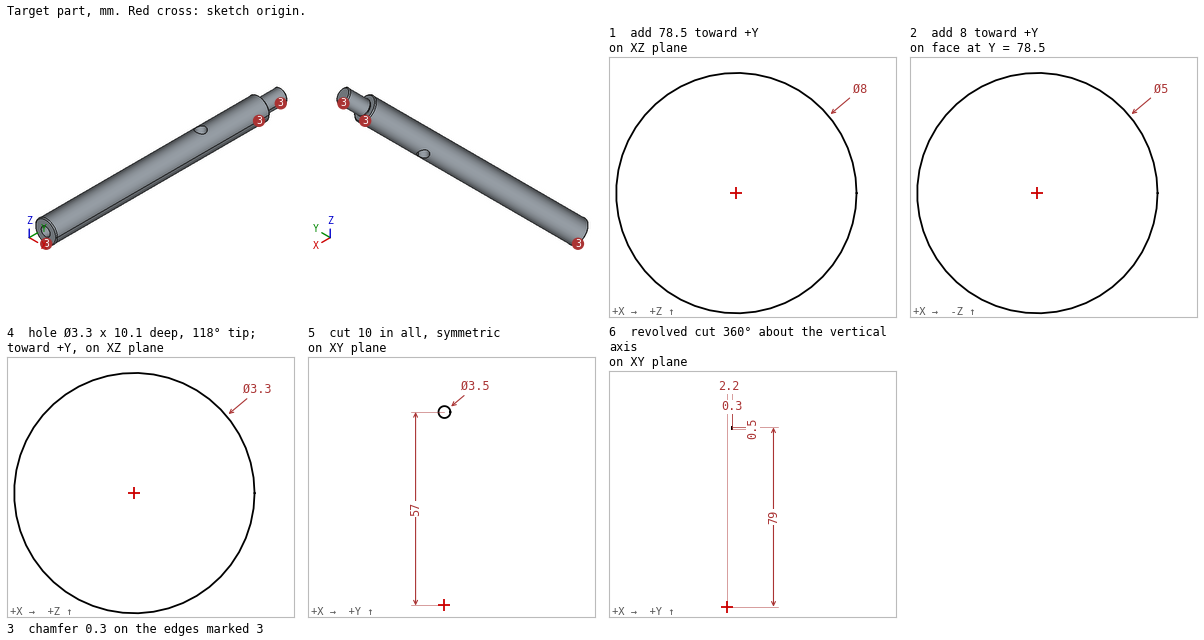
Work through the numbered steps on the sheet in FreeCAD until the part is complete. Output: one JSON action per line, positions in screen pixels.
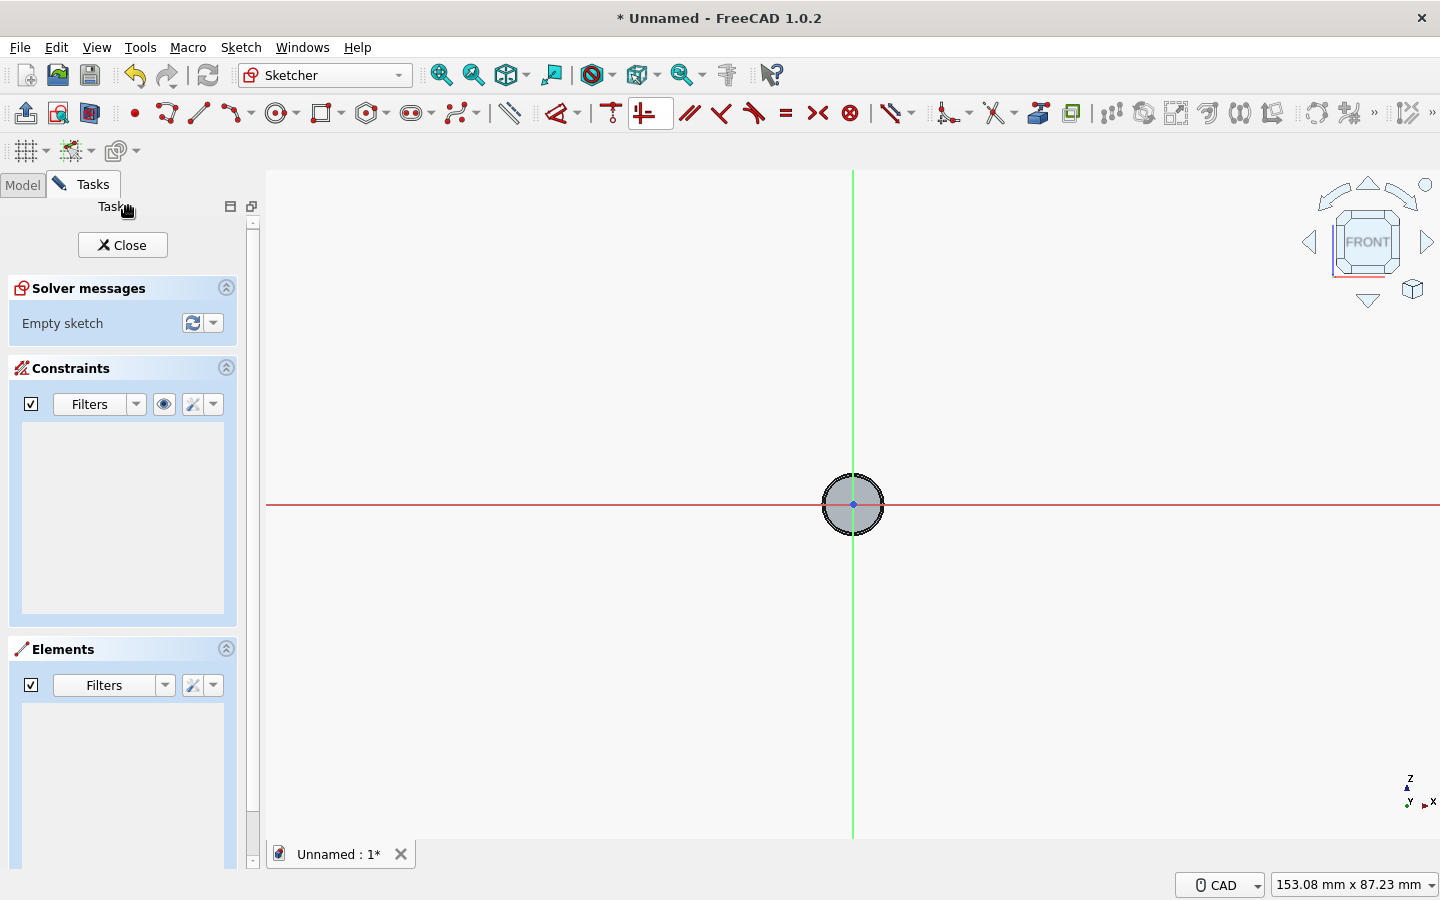
{"action": "scroll", "coordinate": [857, 505], "scroll_direction": "up", "scroll_amount": 14}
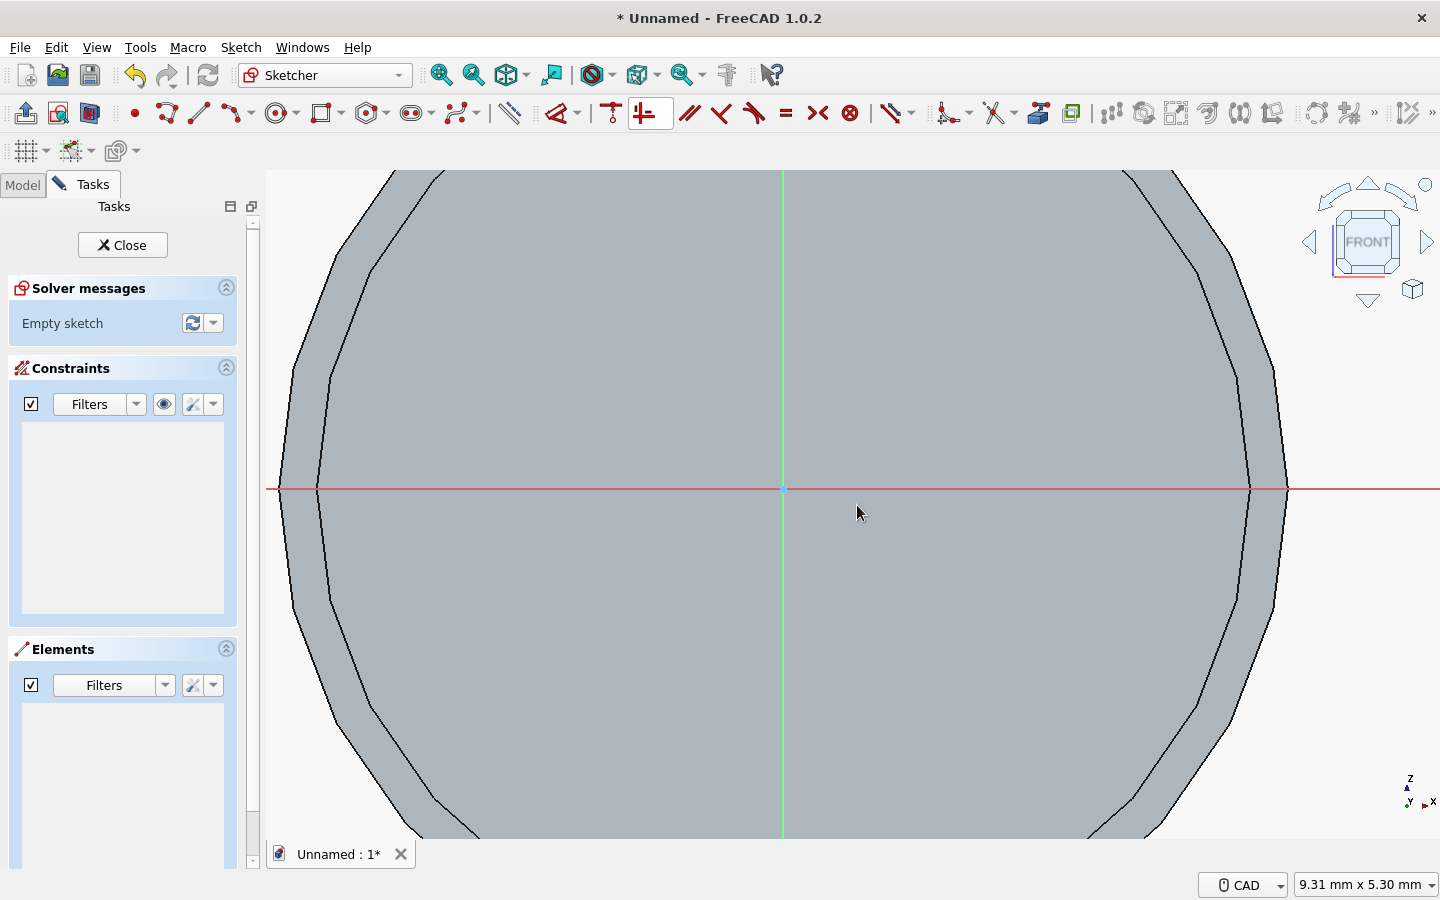
{"action": "key", "text": "g c"}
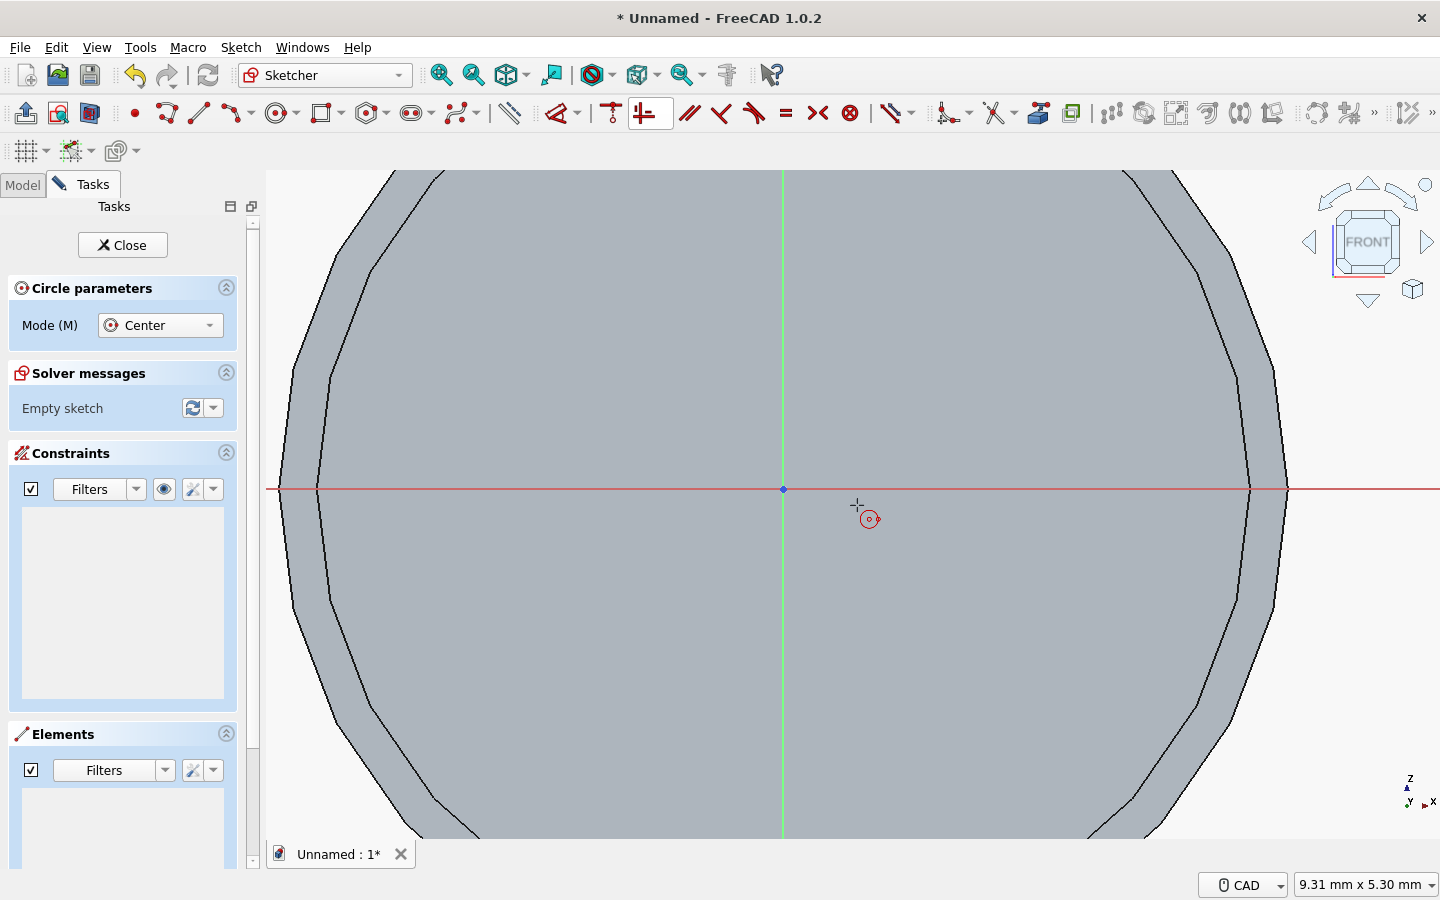
{"action": "left_click", "coordinate": [783, 489]}
{"action": "left_click", "coordinate": [931, 342]}
{"action": "key", "text": "Escape"}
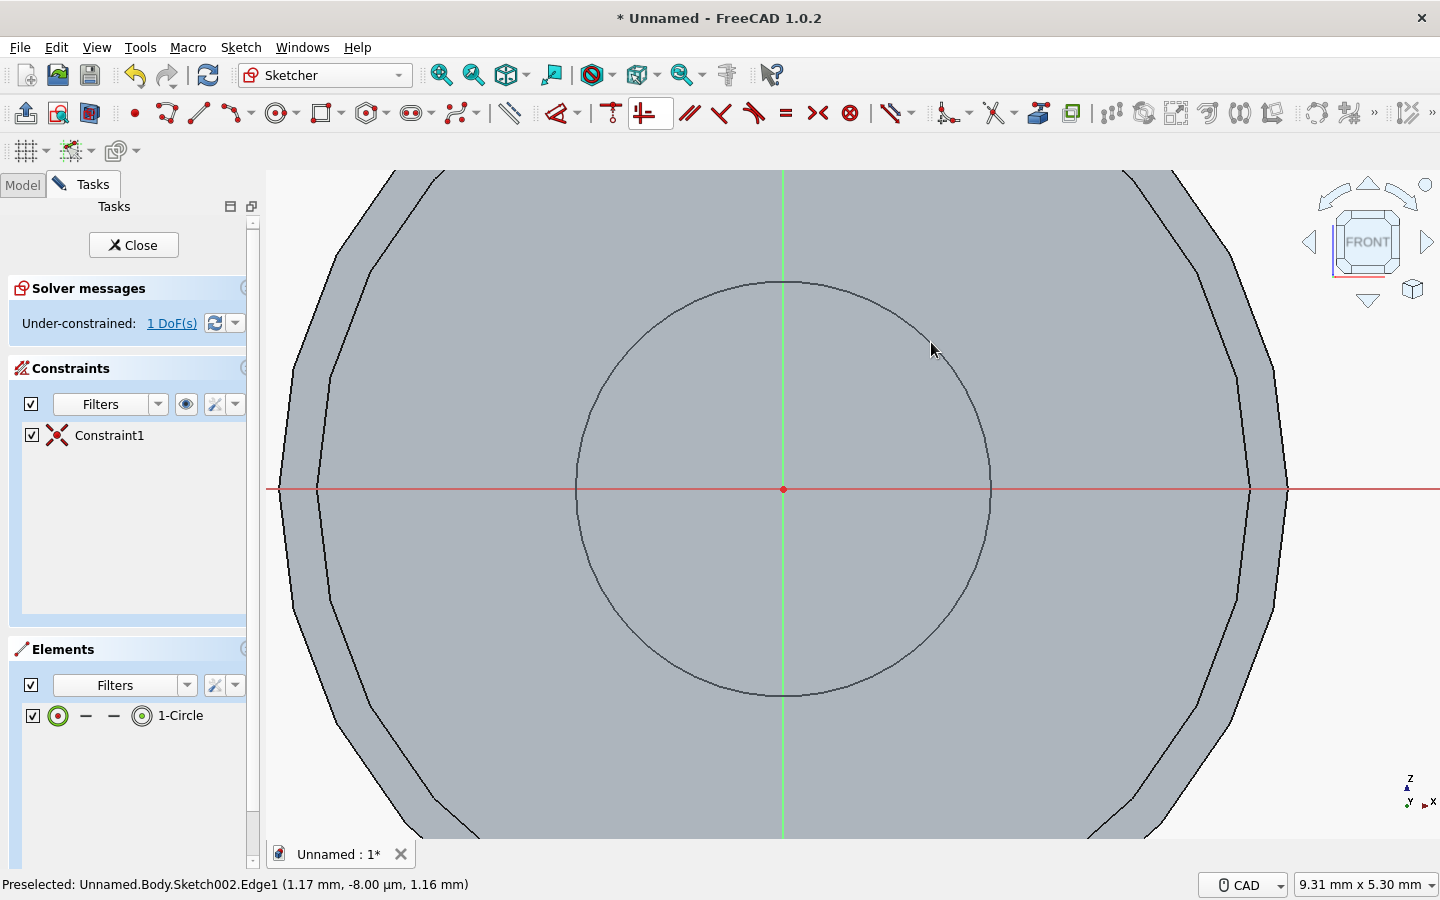
{"action": "key", "text": "d"}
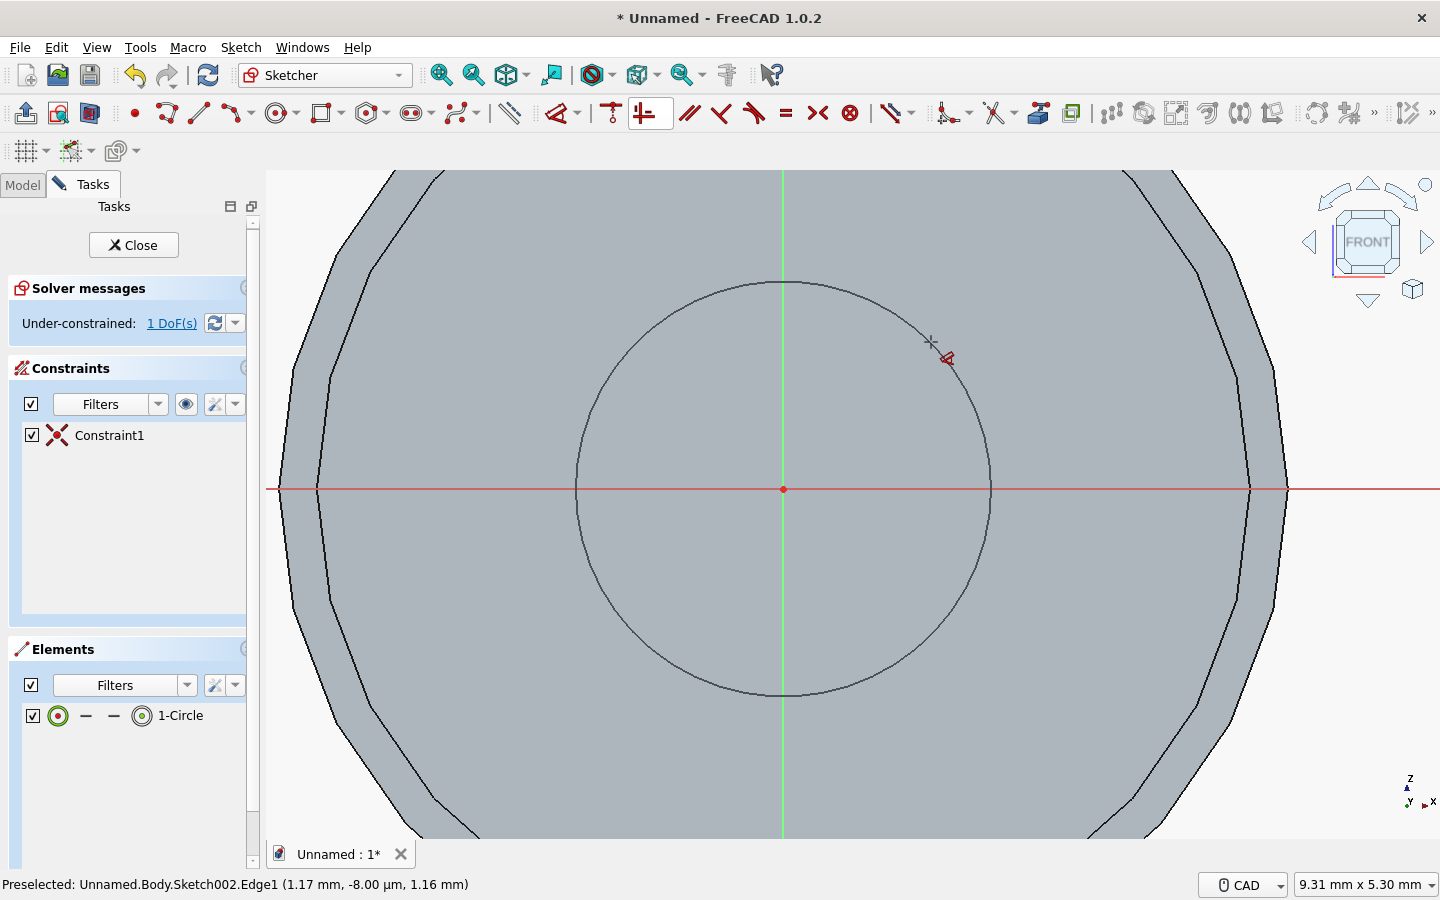
{"action": "left_click", "coordinate": [930, 342]}
{"action": "left_click", "coordinate": [953, 319]}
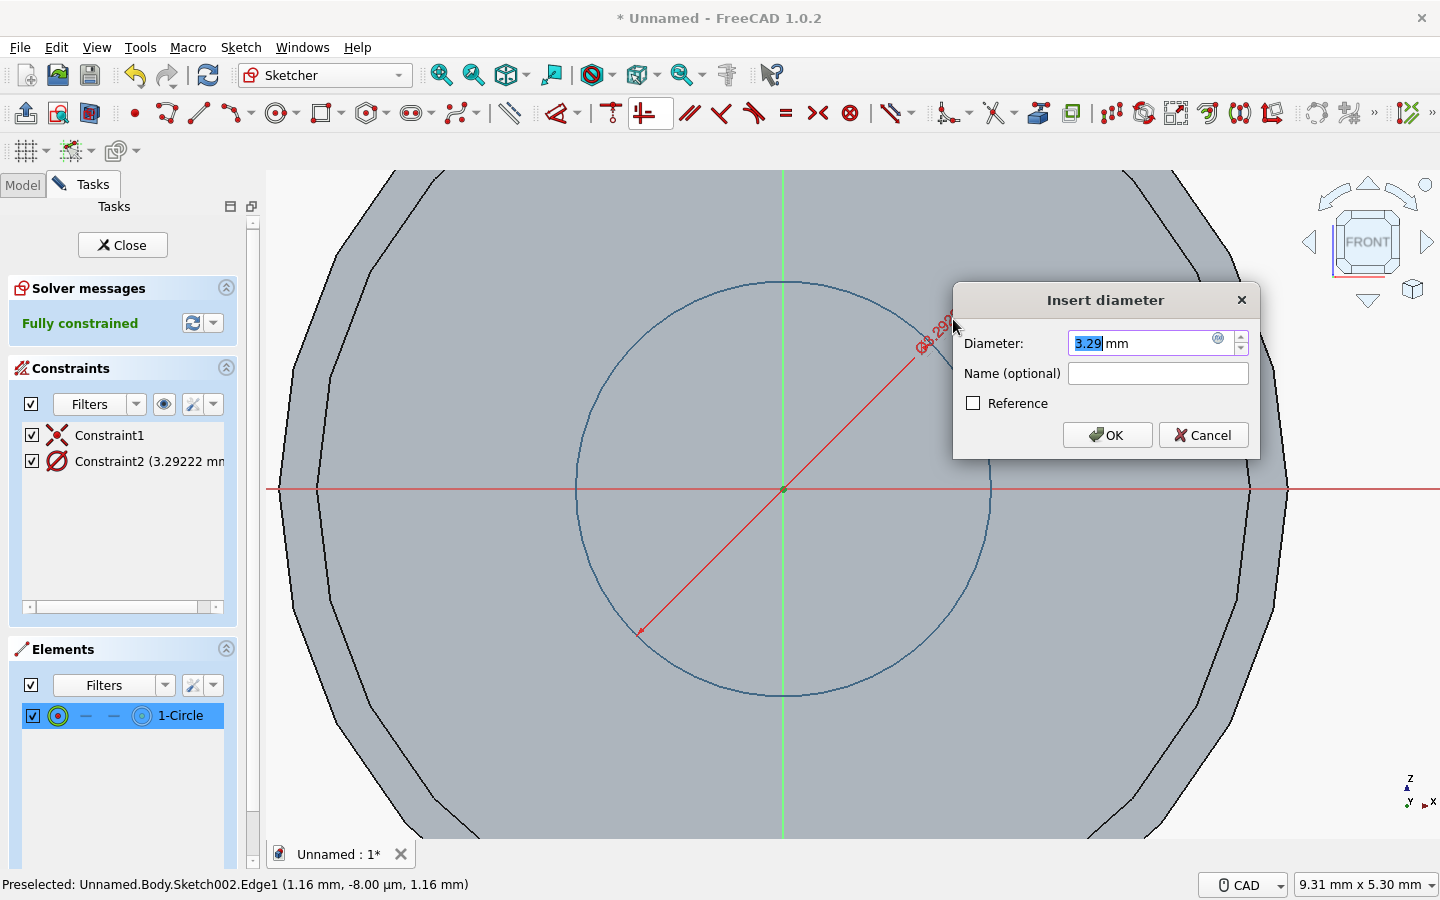
{"action": "type", "text": "3.3"}
{"action": "key", "text": "Return"}
{"action": "key", "text": "Escape"}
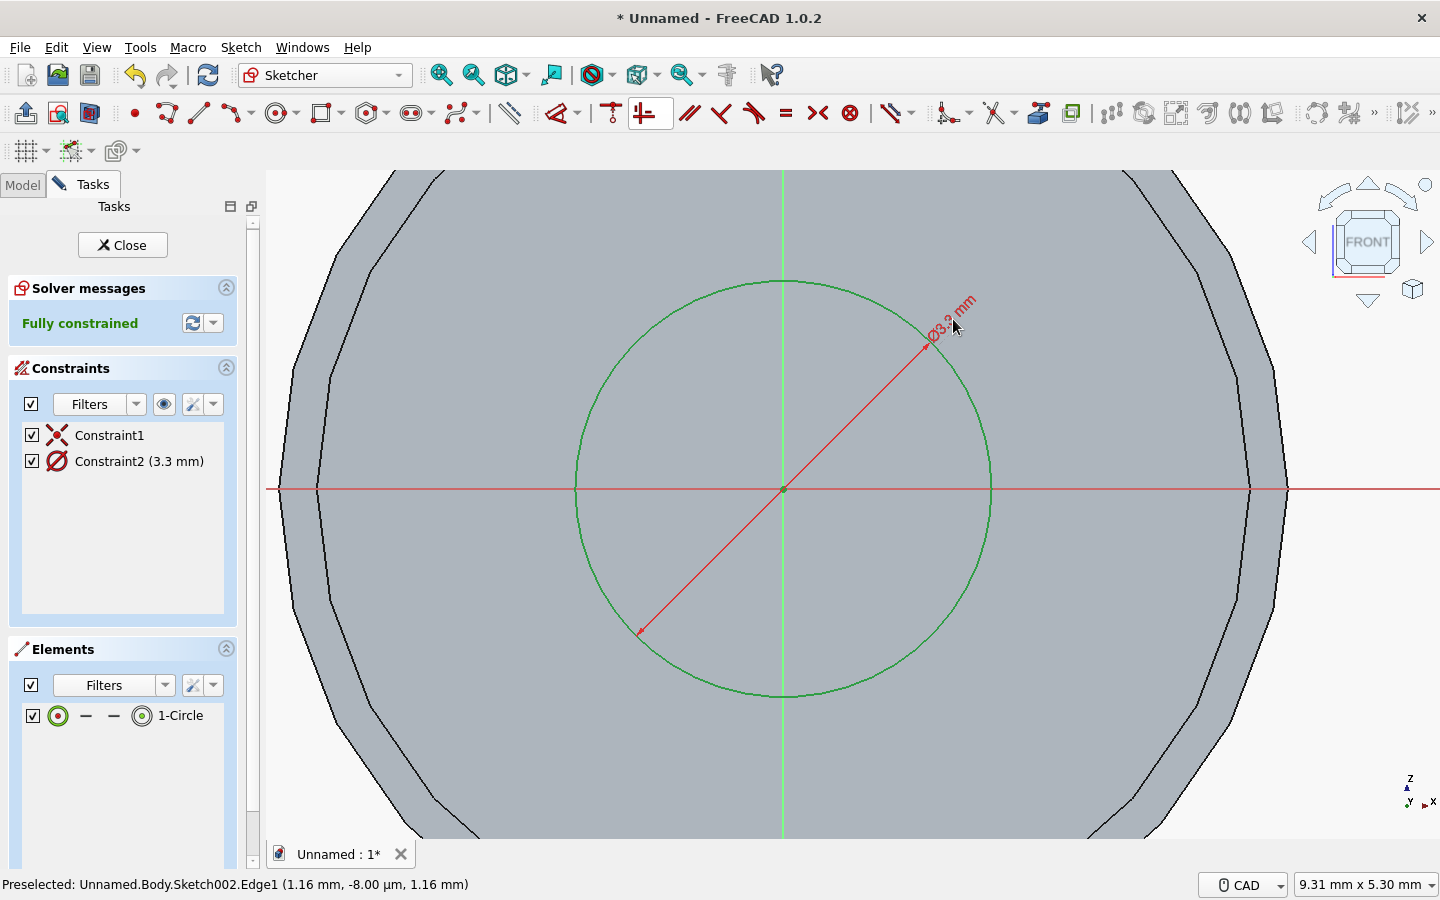
{"action": "left_click", "coordinate": [123, 245]}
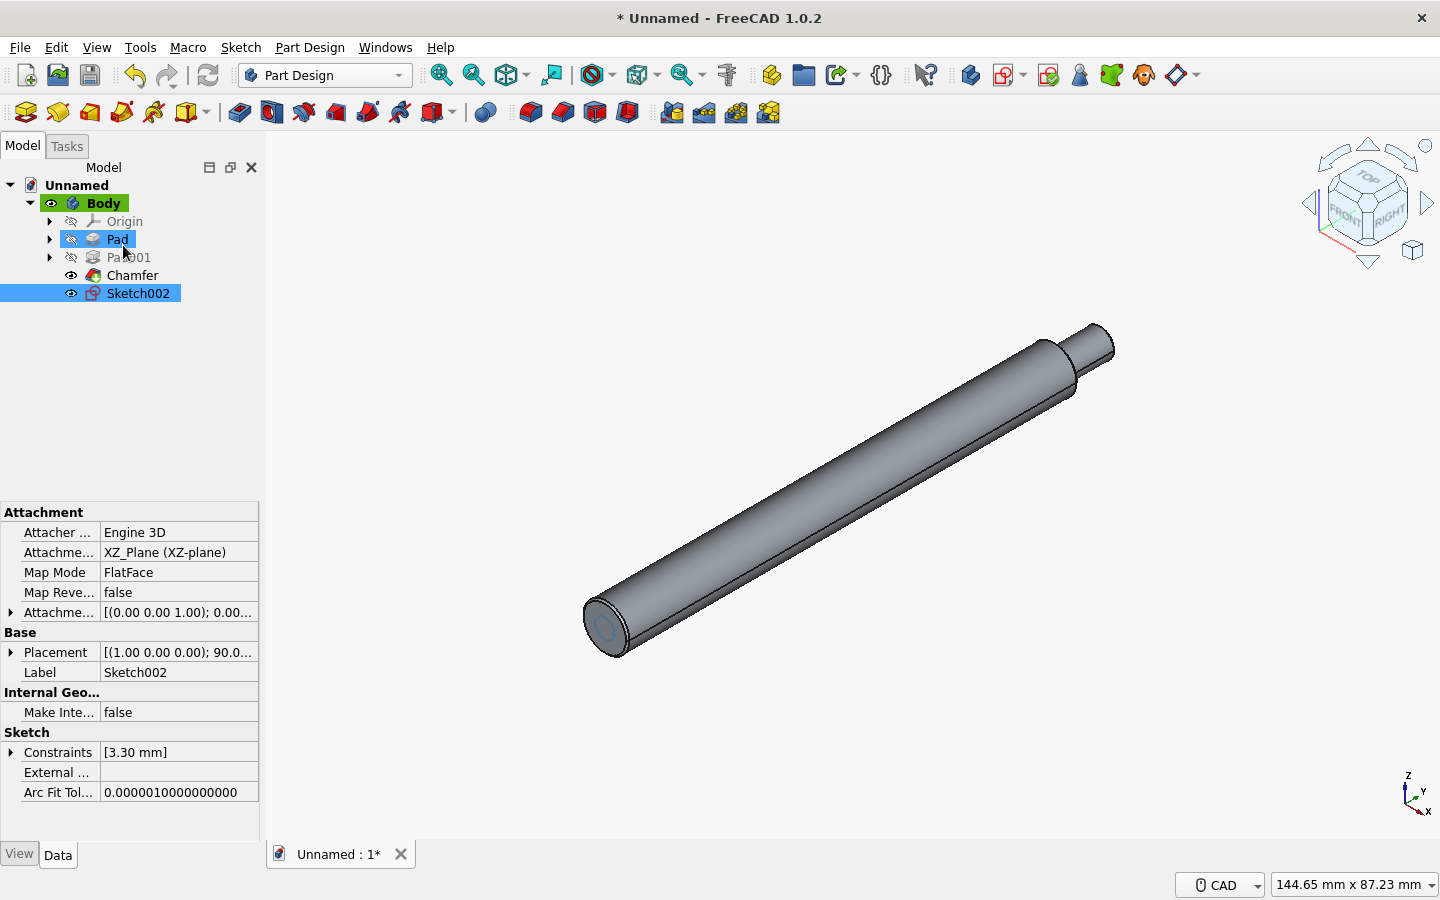
{"action": "left_click", "coordinate": [272, 112]}